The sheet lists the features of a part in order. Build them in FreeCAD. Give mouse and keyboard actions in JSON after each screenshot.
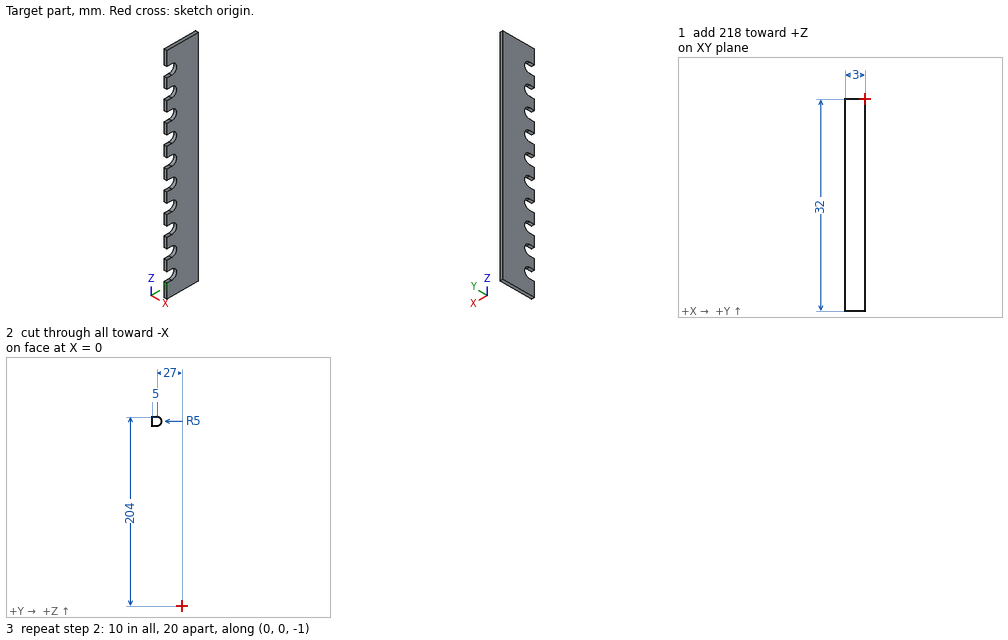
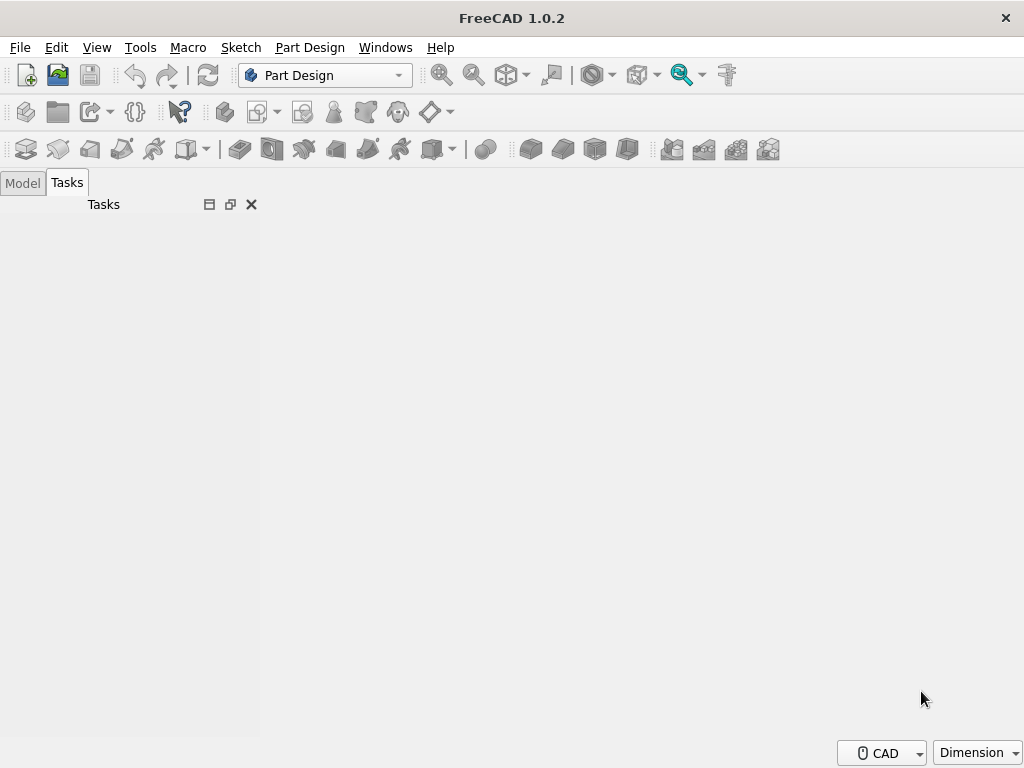
{"action": "left_click", "coordinate": [26, 76]}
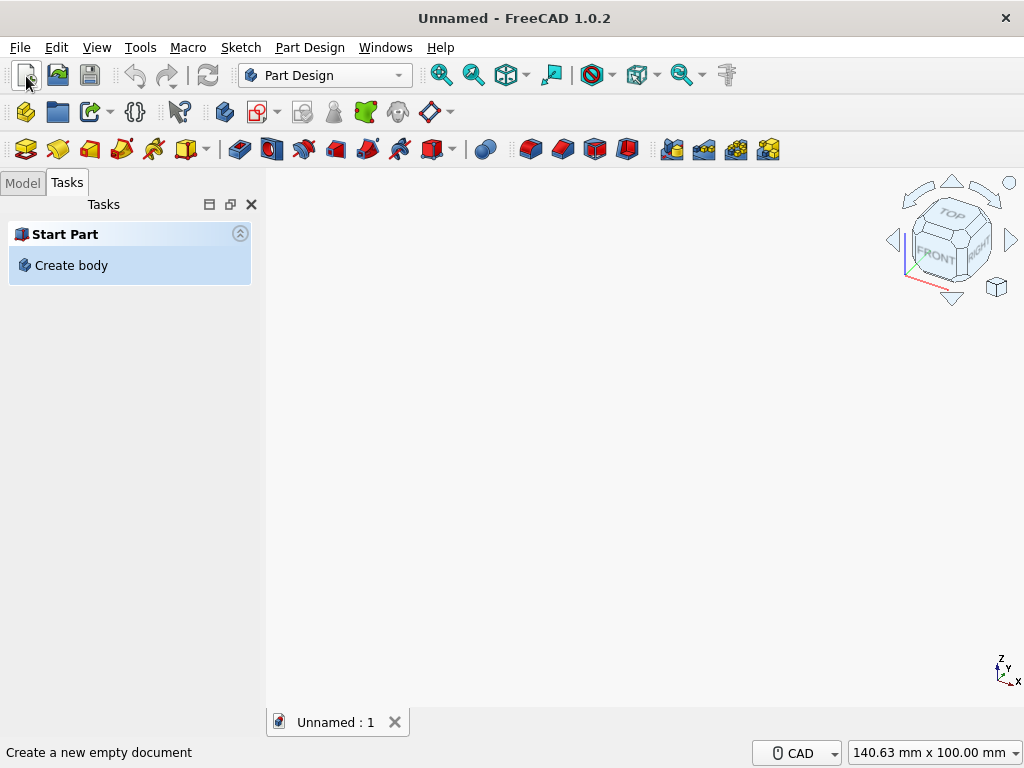
{"action": "left_click", "coordinate": [258, 112]}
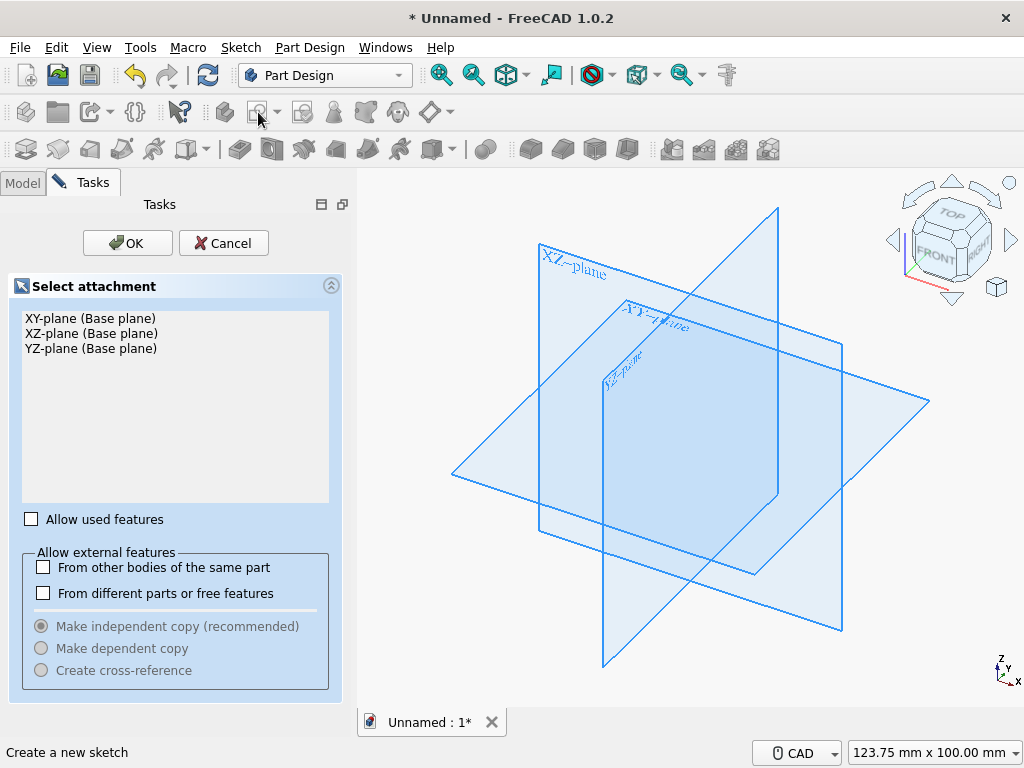
{"action": "left_click", "coordinate": [82, 318]}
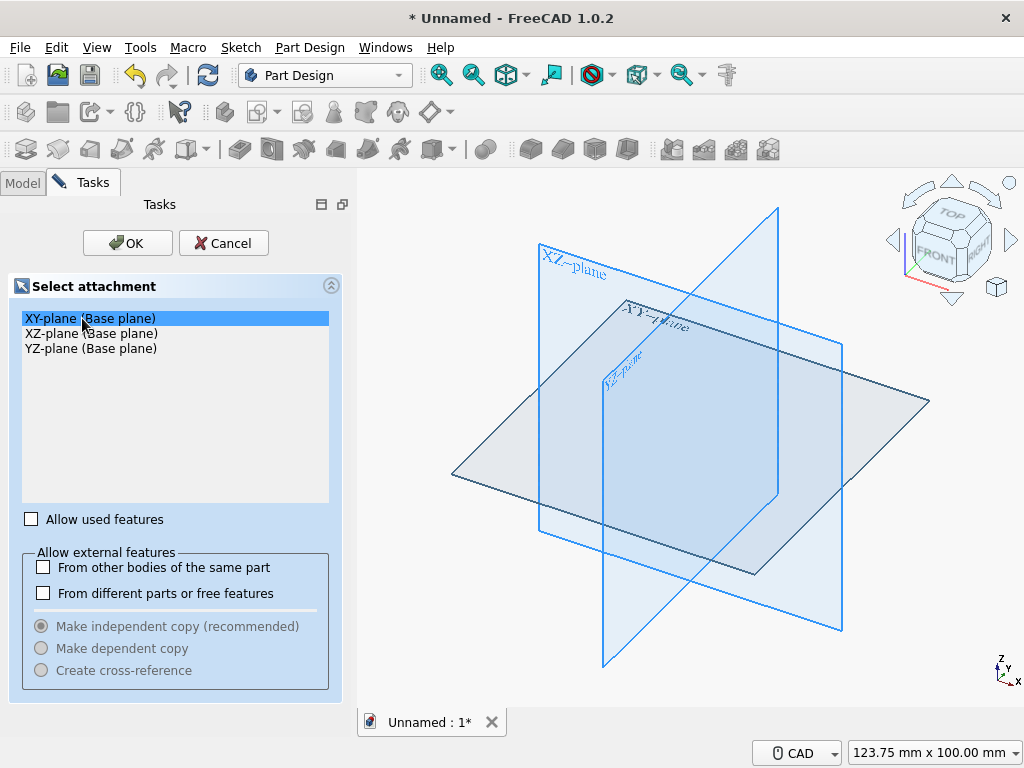
{"action": "left_click", "coordinate": [128, 243]}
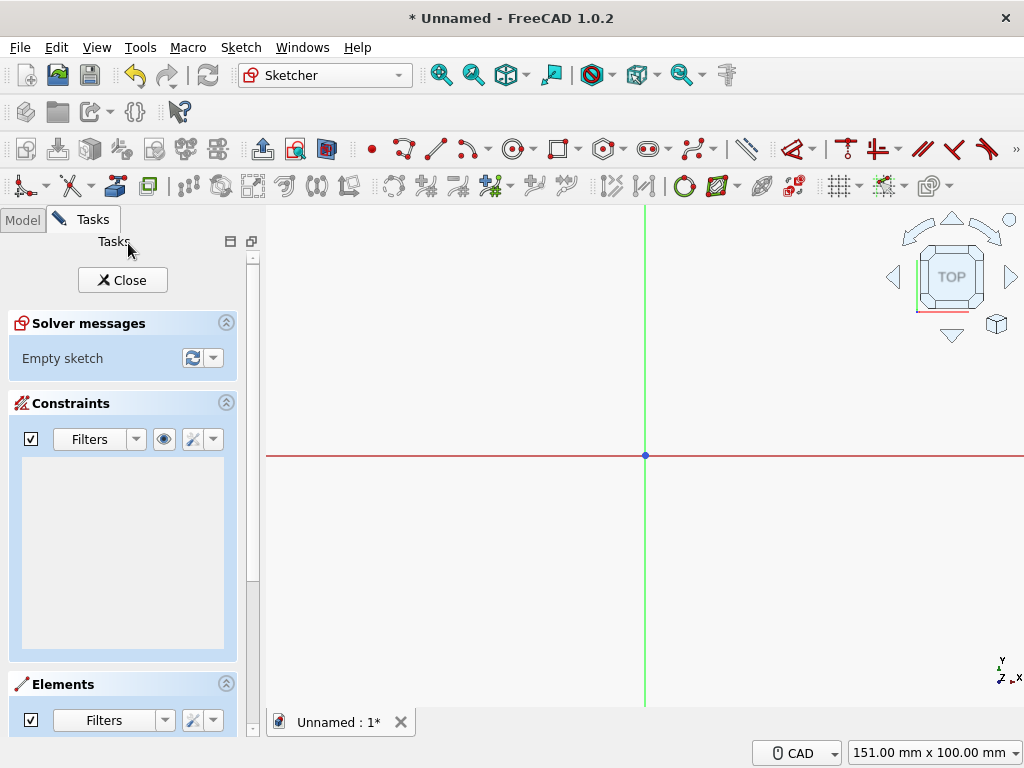
{"action": "scroll", "coordinate": [712, 634], "scroll_direction": "up", "scroll_amount": 3}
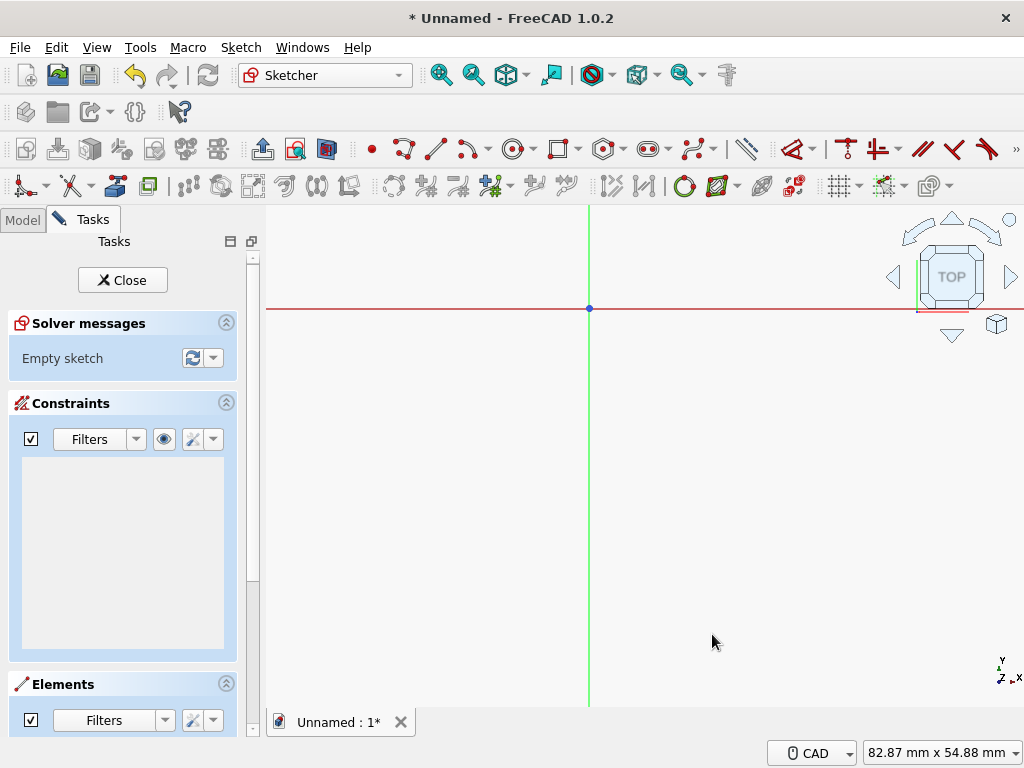
{"action": "left_click", "coordinate": [558, 150]}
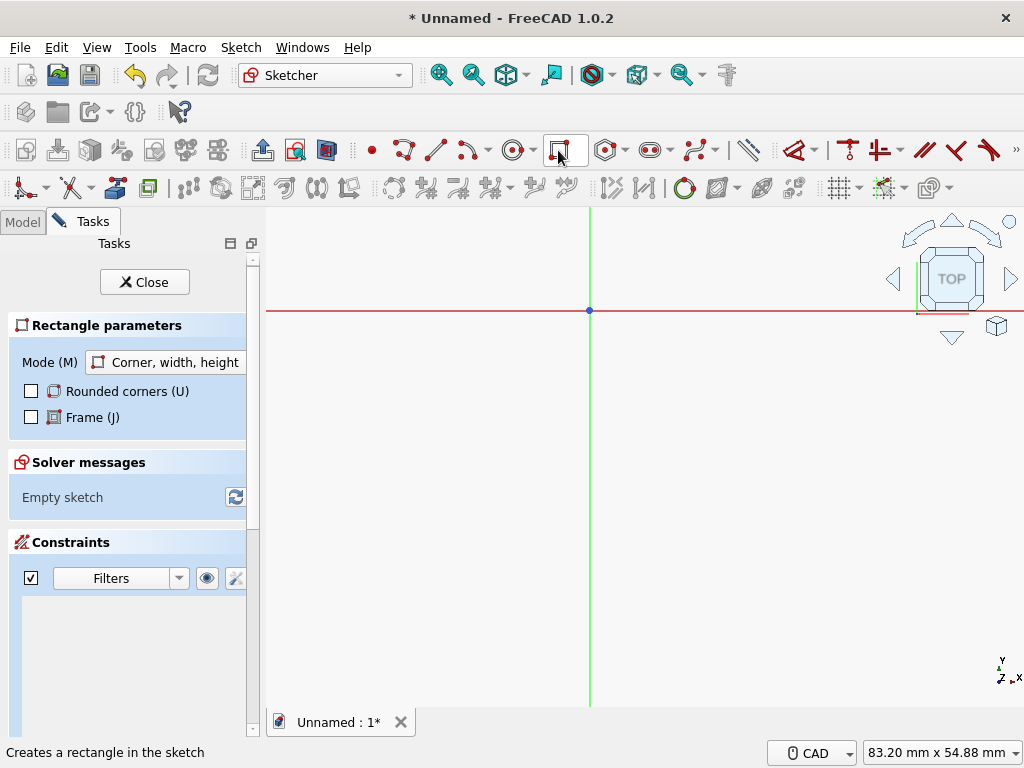
{"action": "left_click", "coordinate": [590, 311]}
{"action": "left_click", "coordinate": [562, 602]}
{"action": "key", "text": "Escape"}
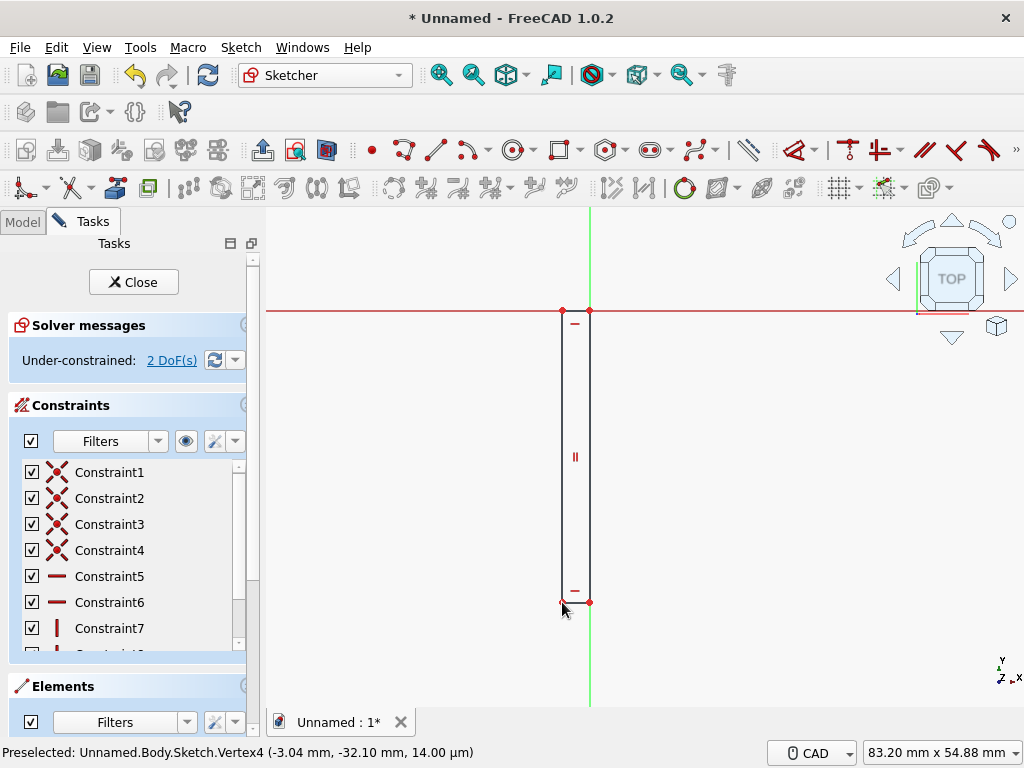
{"action": "left_click", "coordinate": [794, 150]}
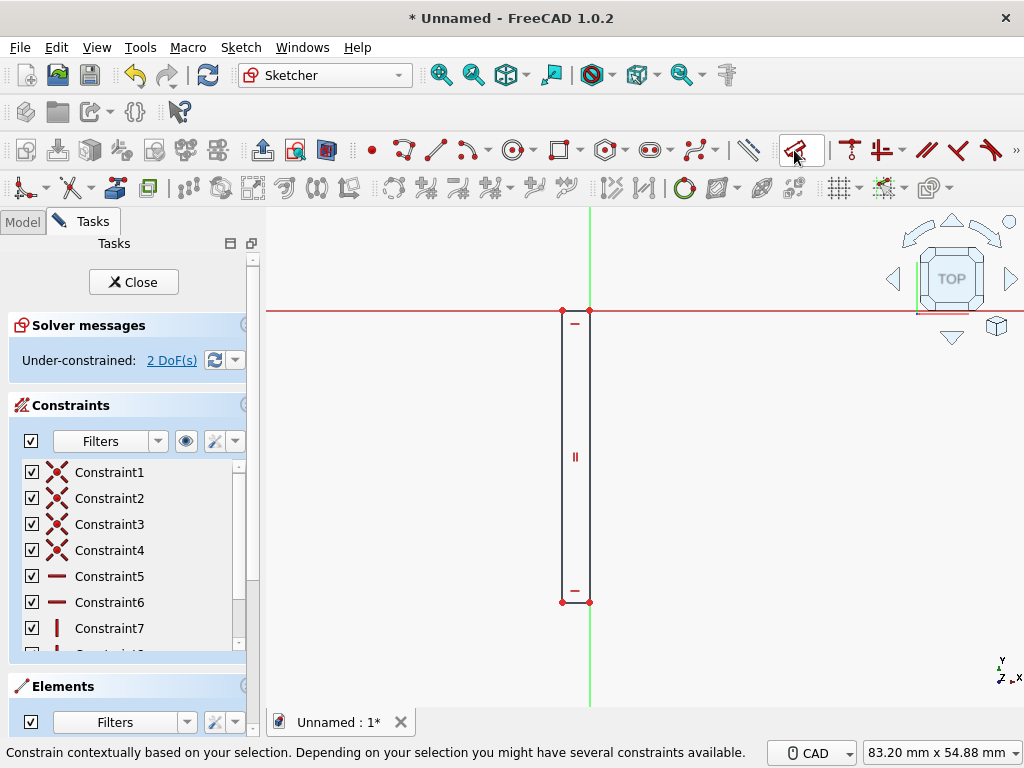
{"action": "scroll", "coordinate": [579, 311], "scroll_direction": "up", "scroll_amount": 2}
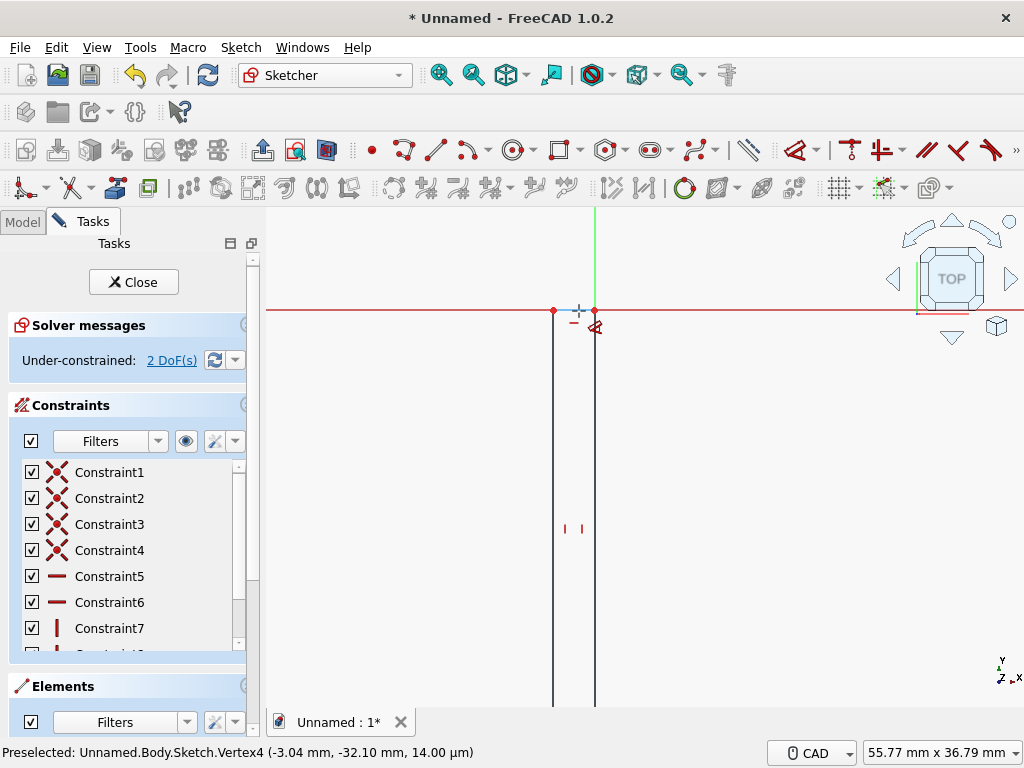
{"action": "left_click", "coordinate": [578, 310]}
{"action": "left_click", "coordinate": [574, 276]}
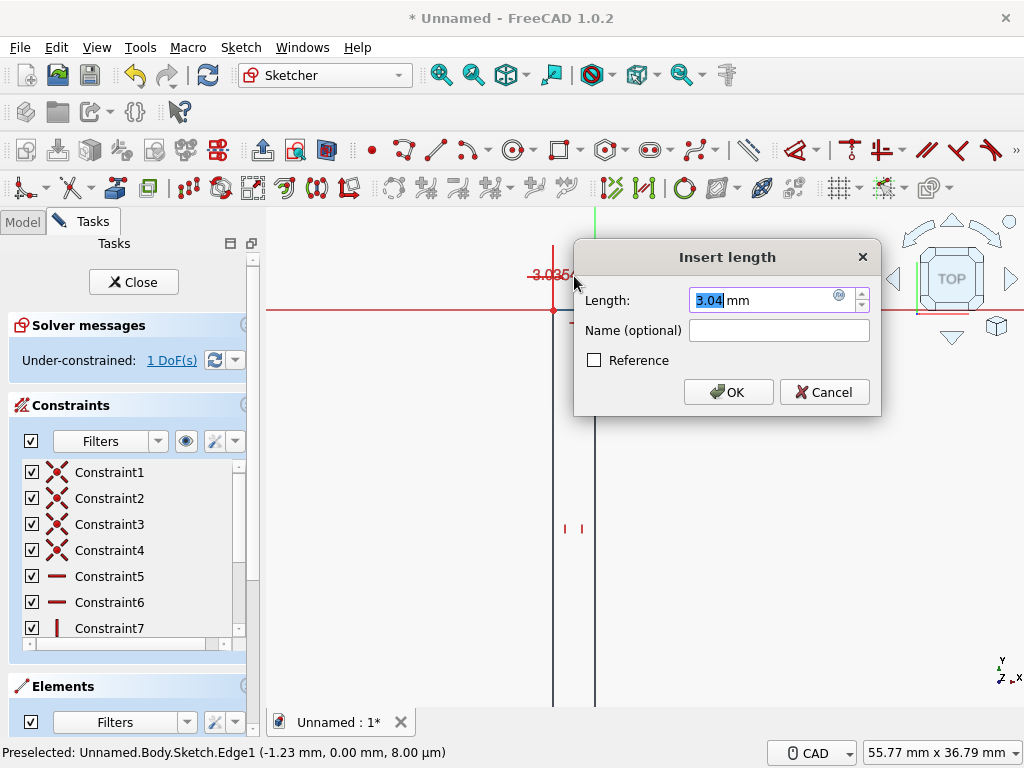
{"action": "type", "text": "3"}
{"action": "key", "text": "Return"}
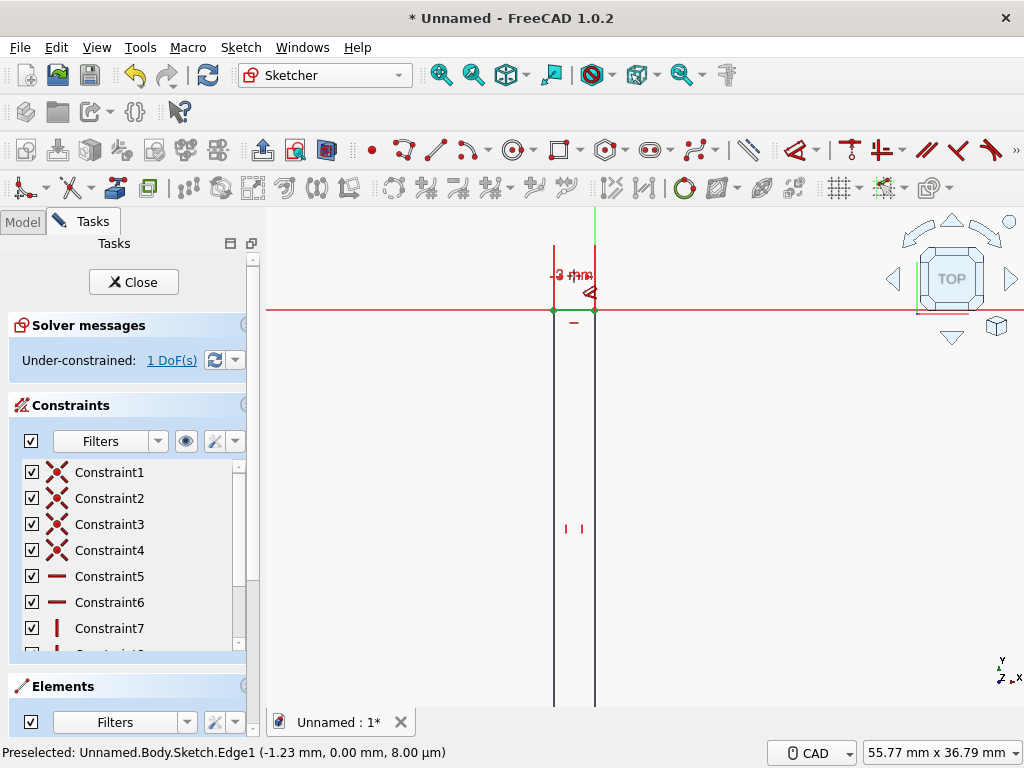
{"action": "left_click", "coordinate": [554, 441]}
{"action": "left_click", "coordinate": [520, 495]}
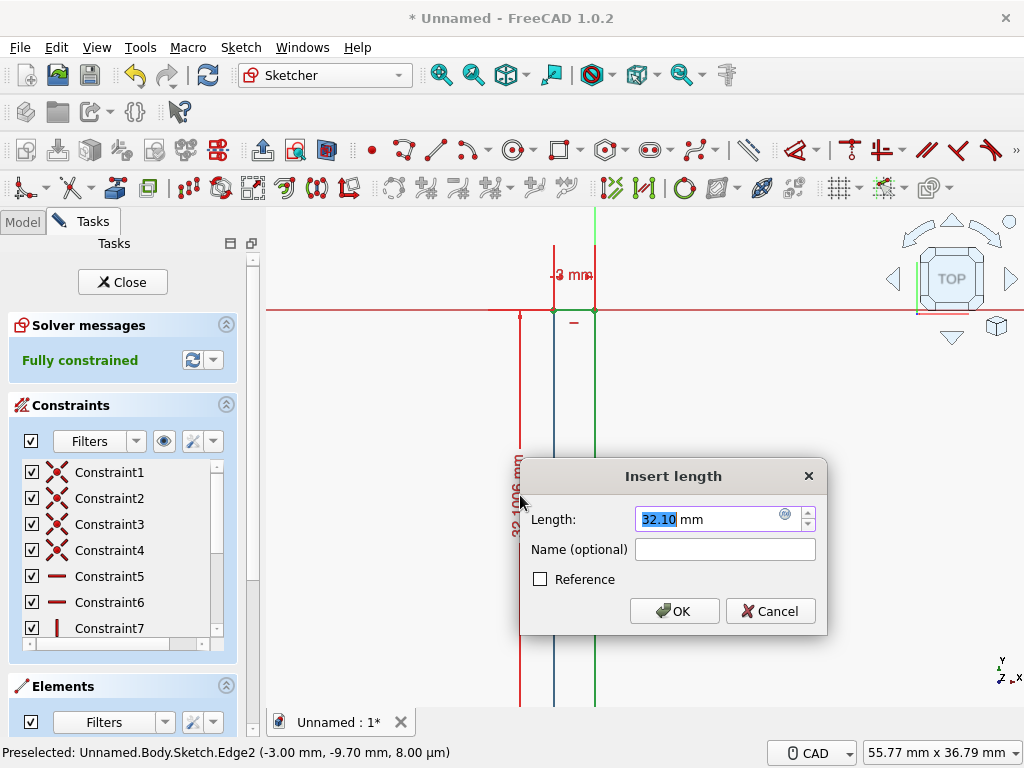
{"action": "type", "text": "32"}
{"action": "key", "text": "Return"}
{"action": "key", "text": "Escape"}